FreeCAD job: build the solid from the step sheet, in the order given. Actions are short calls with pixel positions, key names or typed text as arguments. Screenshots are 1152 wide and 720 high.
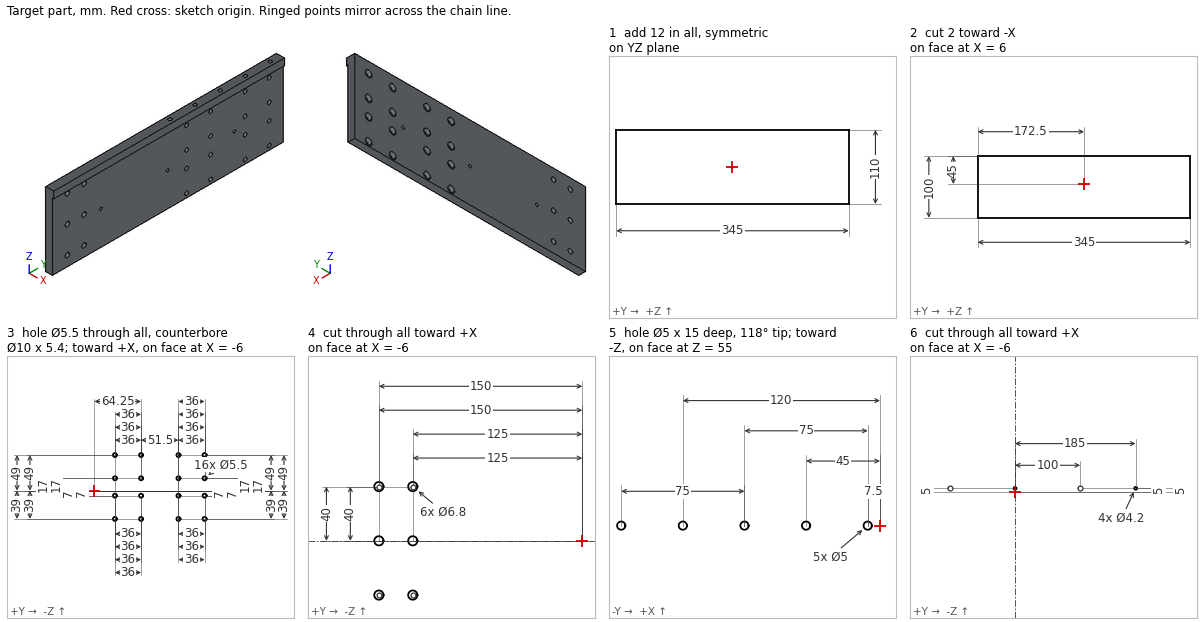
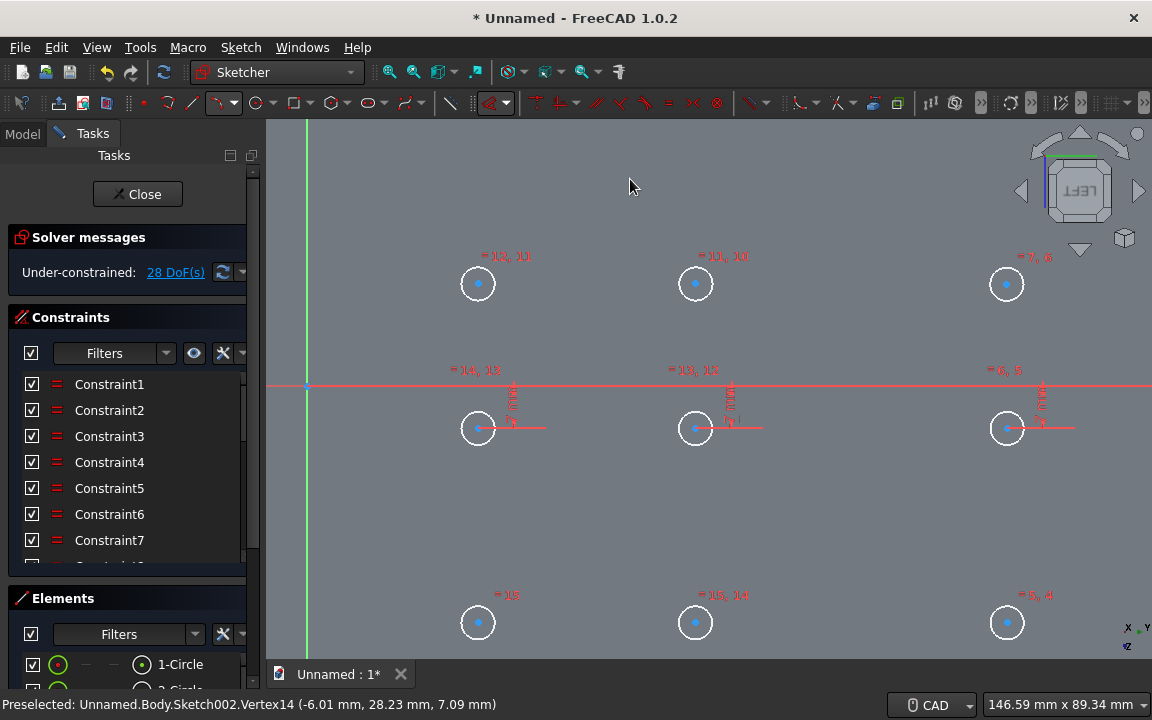
scroll(478, 429, down, 3)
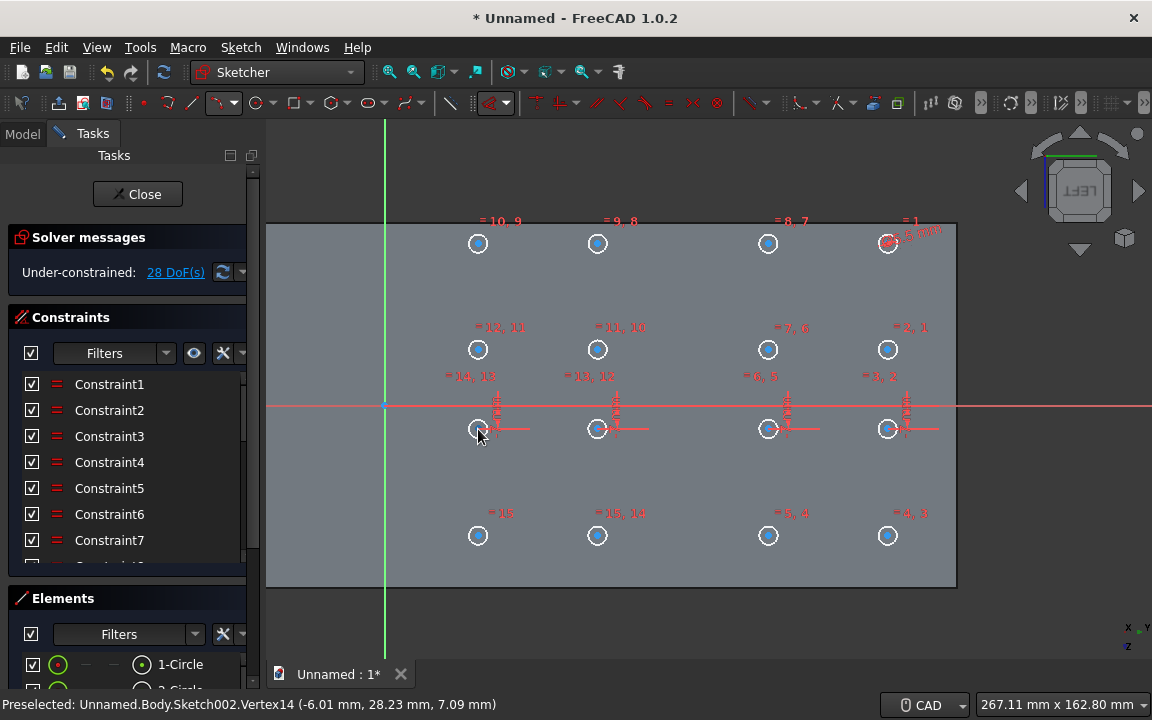
click(888, 244)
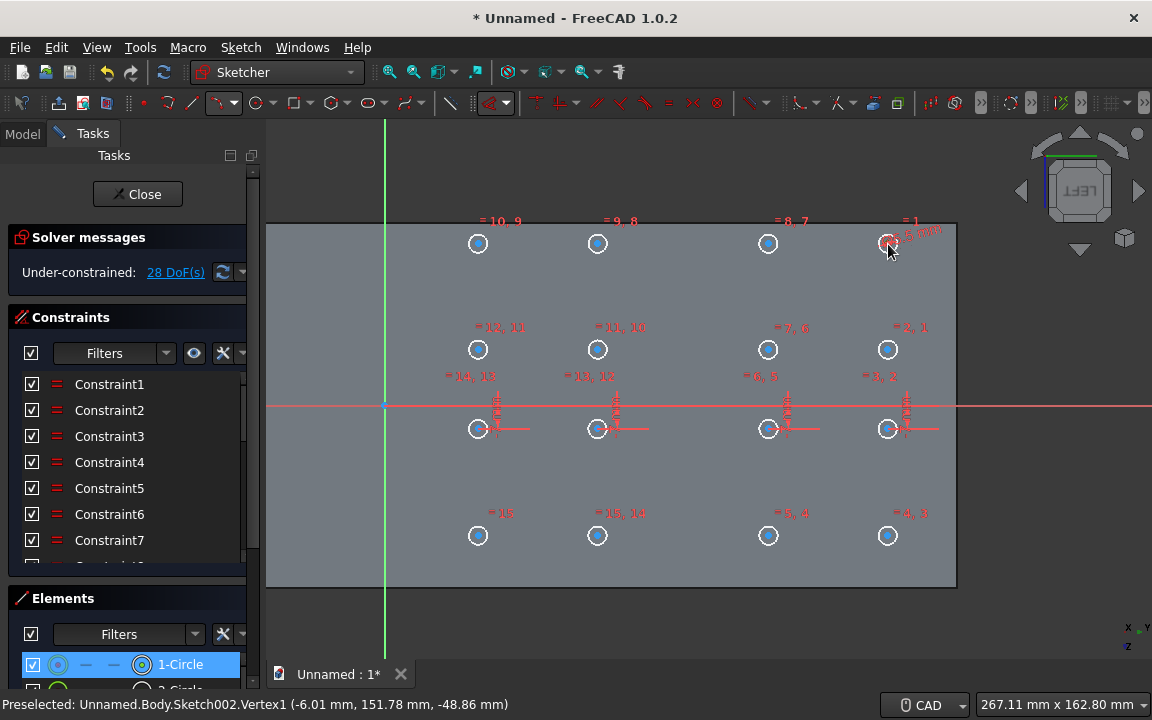
key(i)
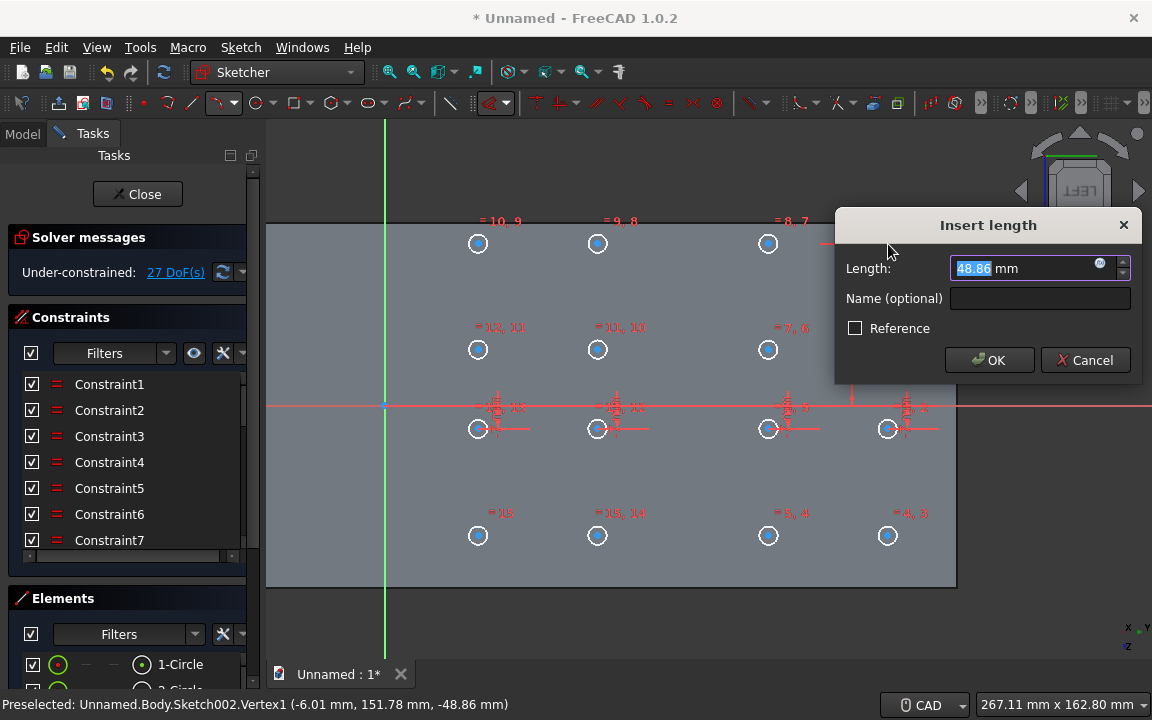
text(49)
key(Return)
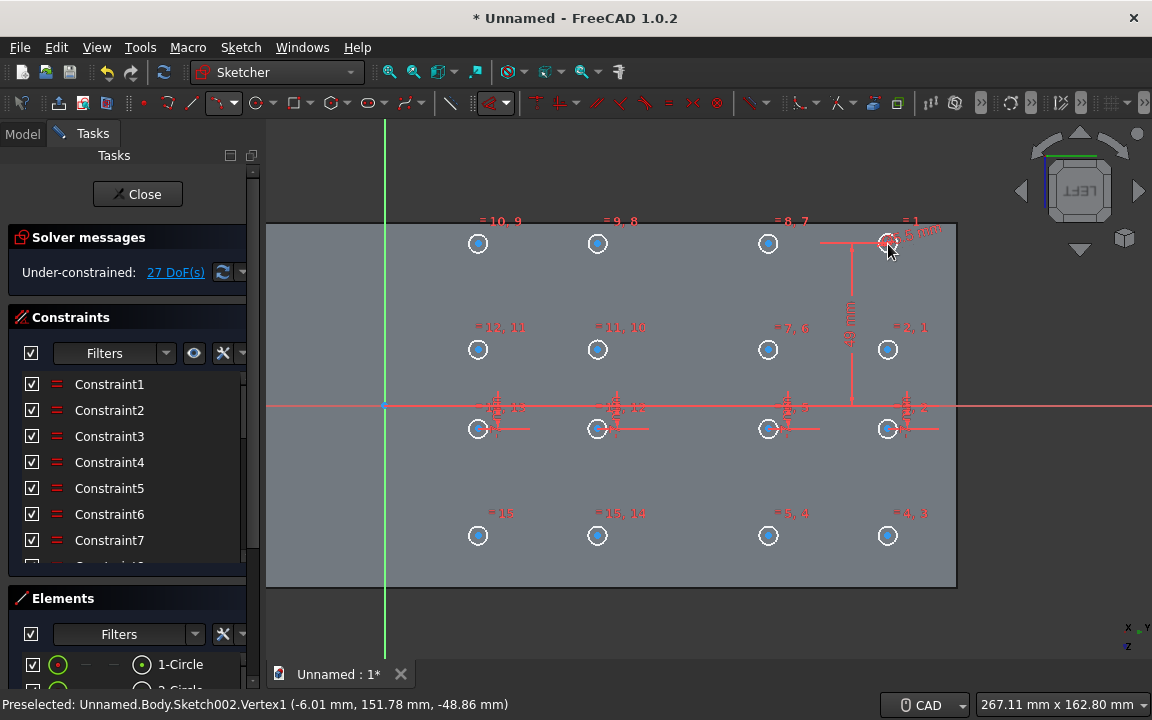
click(888, 350)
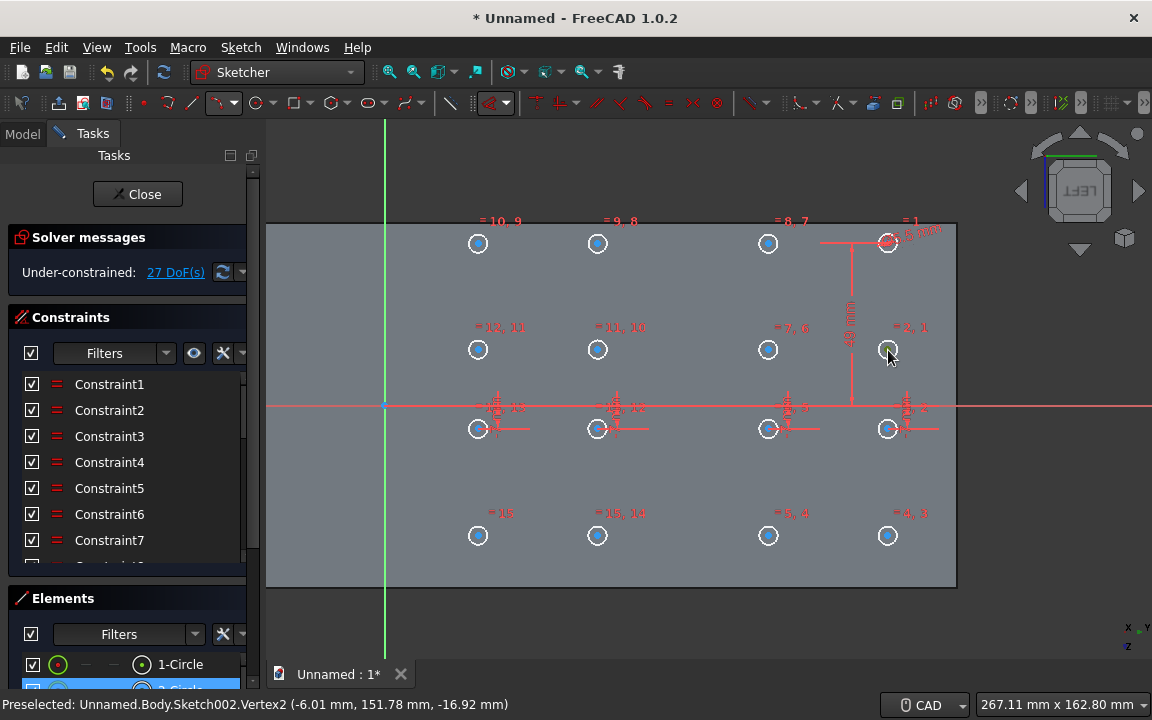
click(508, 104)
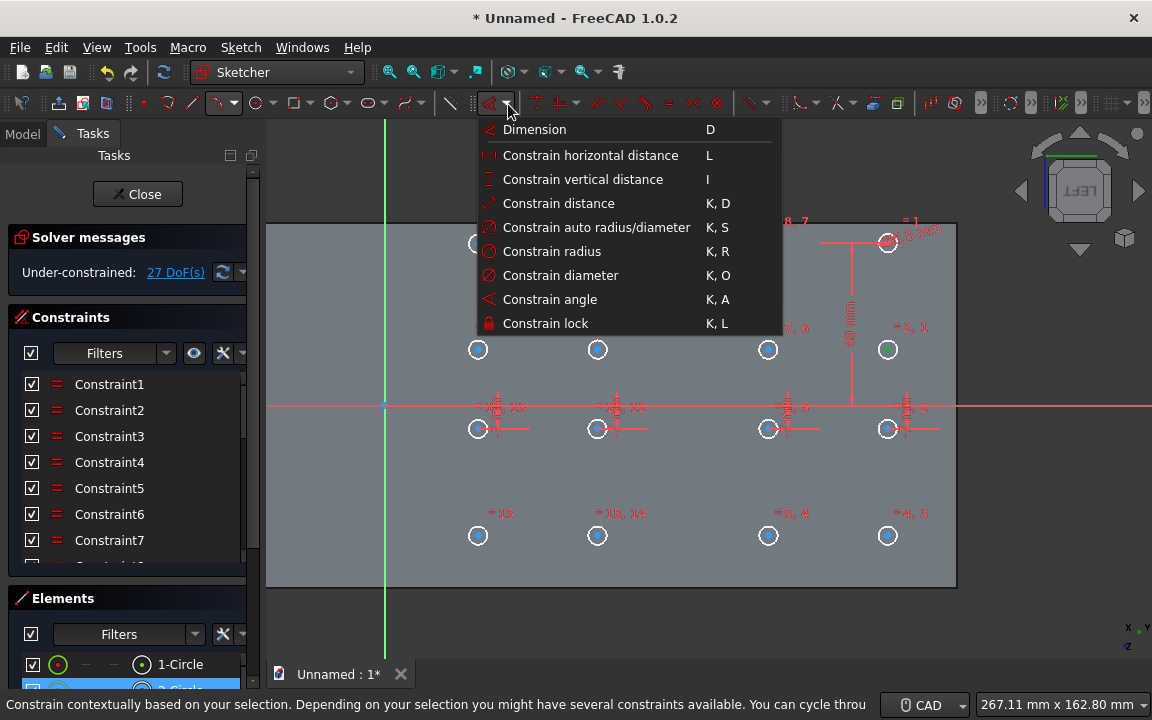
click(630, 179)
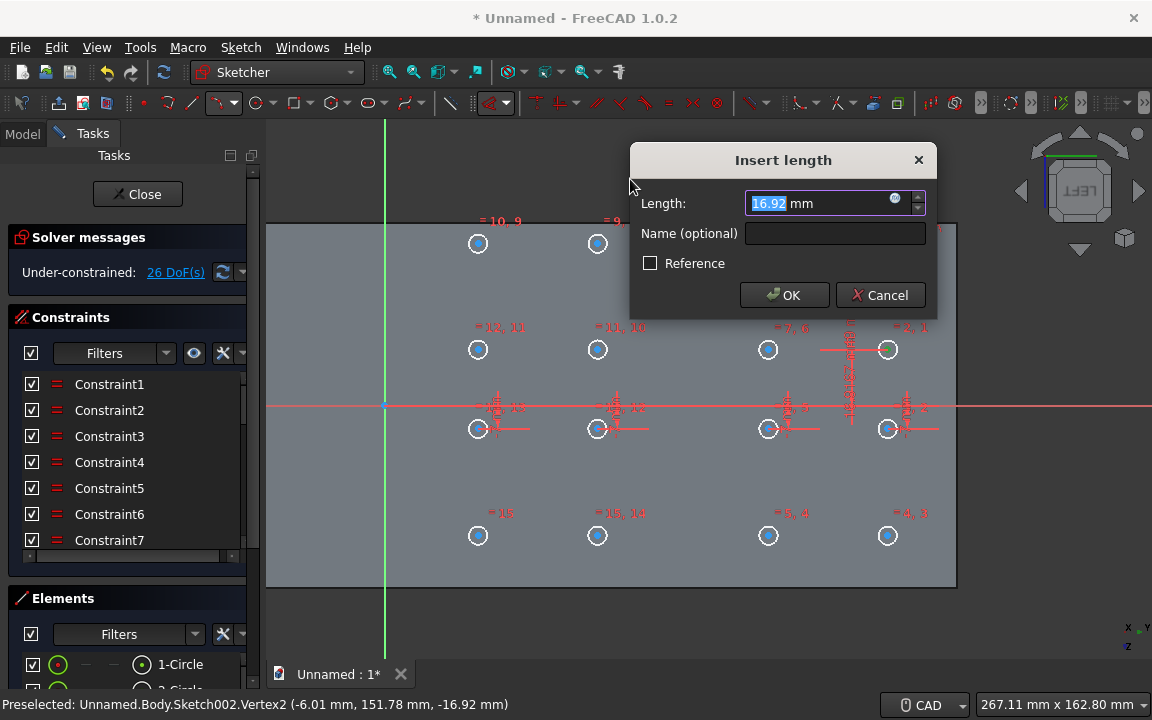
text(17)
key(Return)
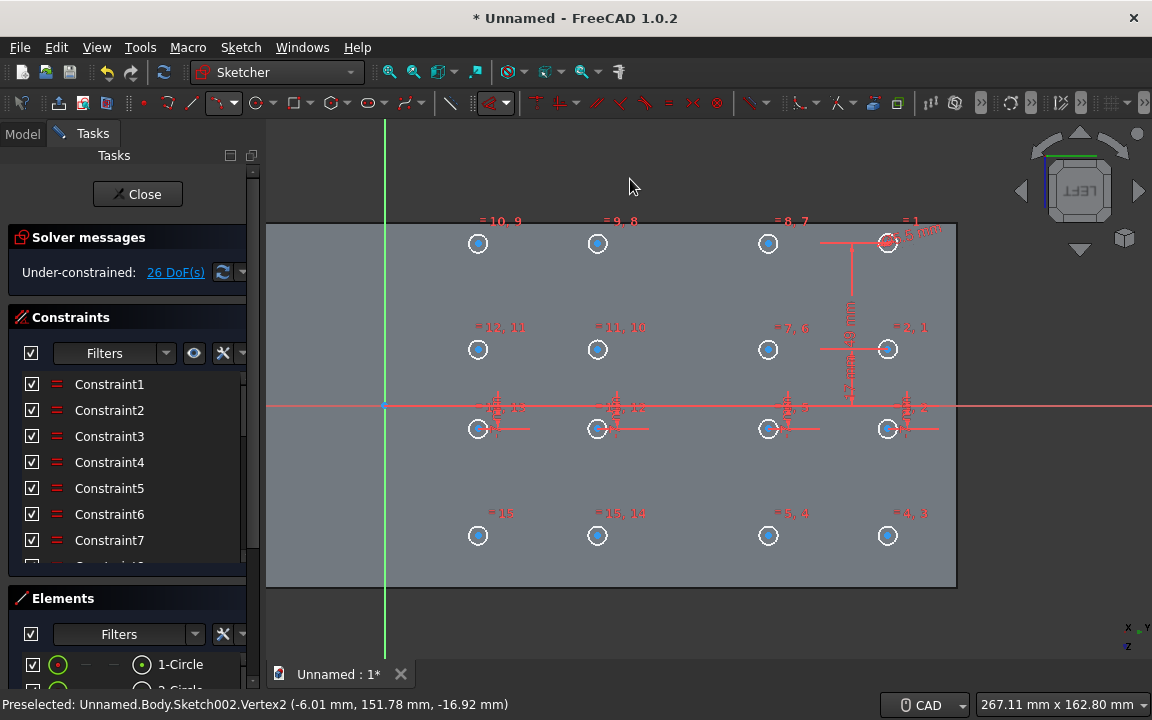
click(888, 536)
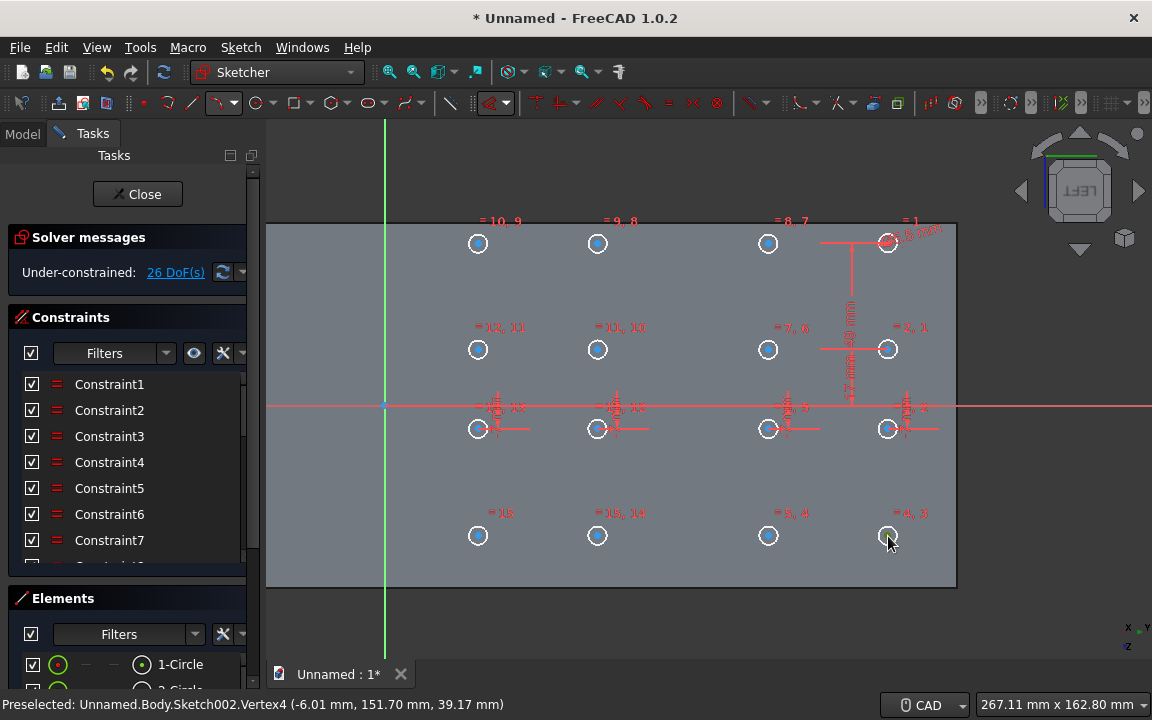
key(i)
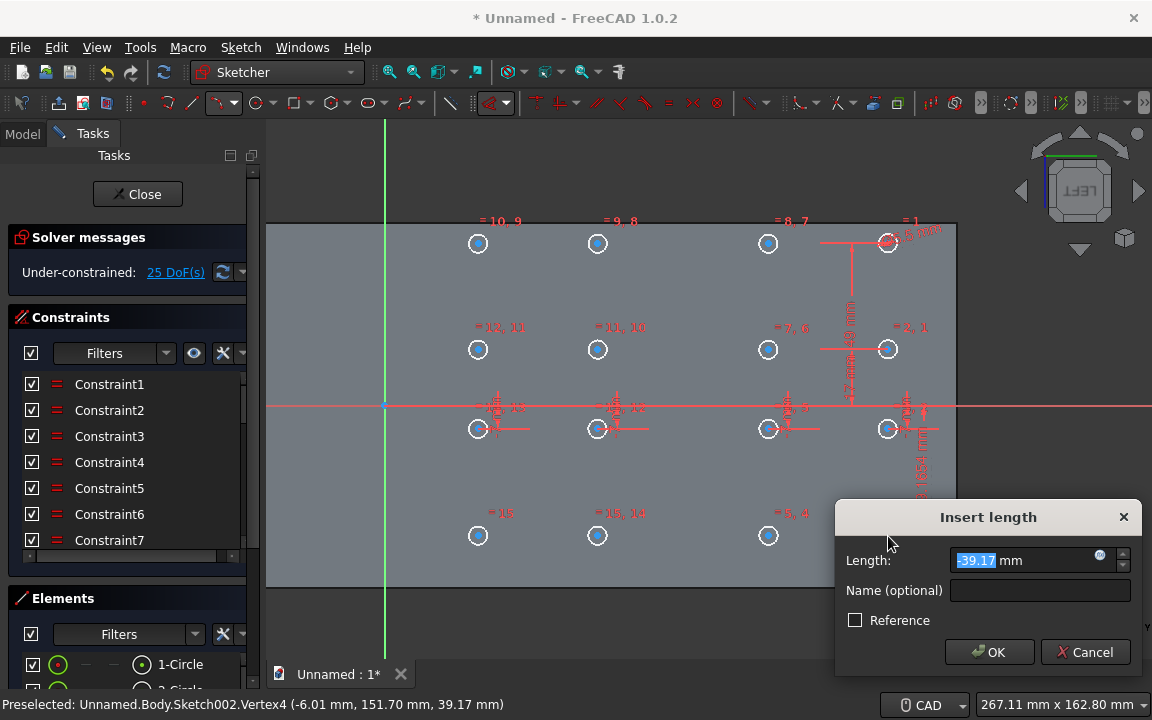
text(-39)
key(Return)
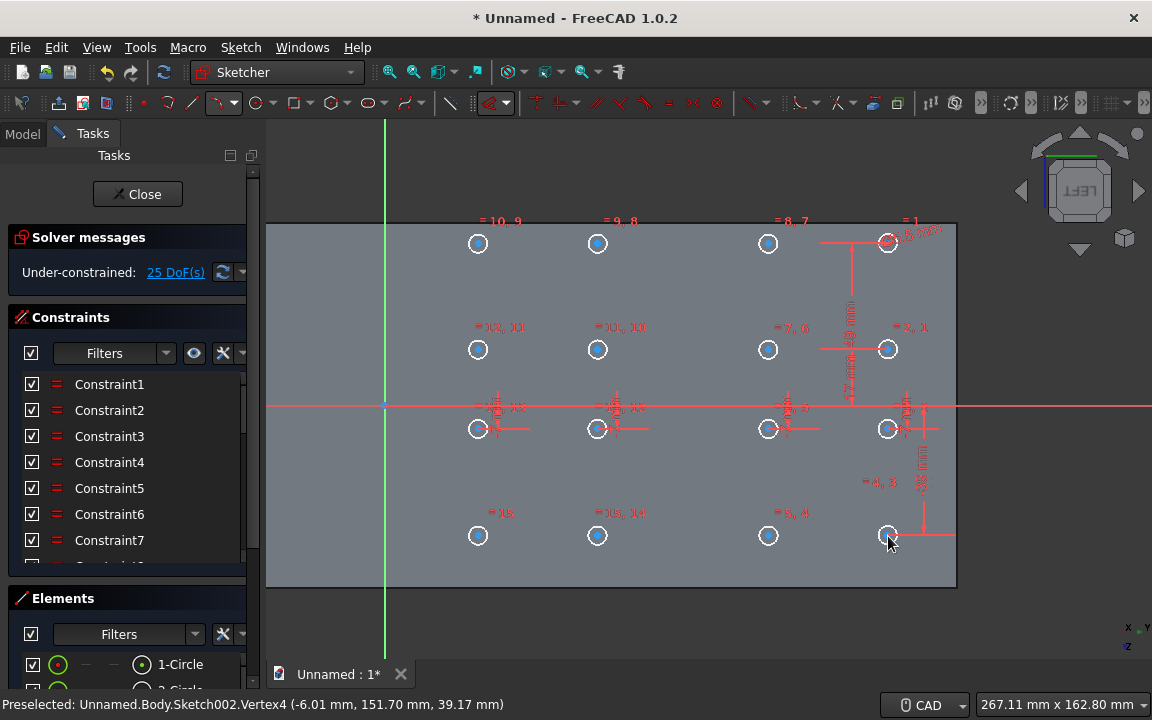
click(769, 536)